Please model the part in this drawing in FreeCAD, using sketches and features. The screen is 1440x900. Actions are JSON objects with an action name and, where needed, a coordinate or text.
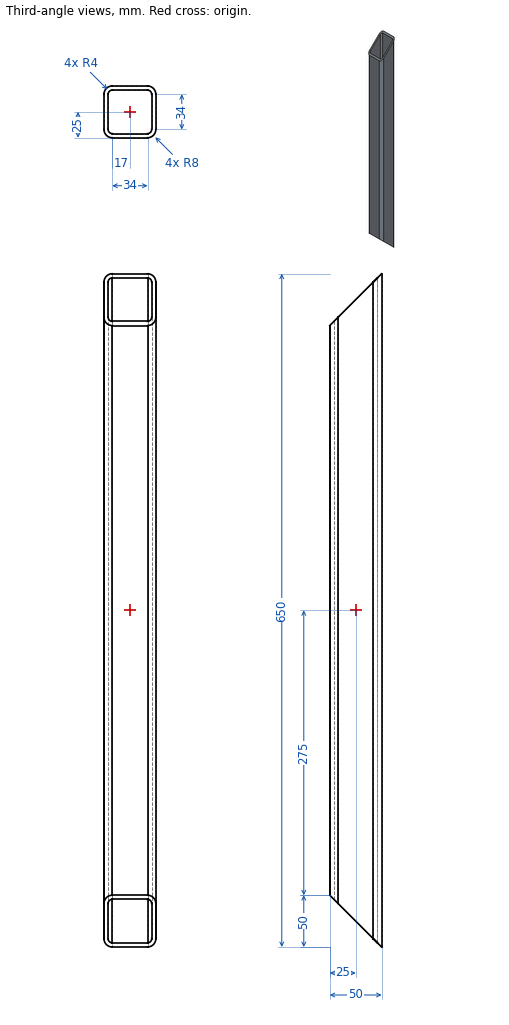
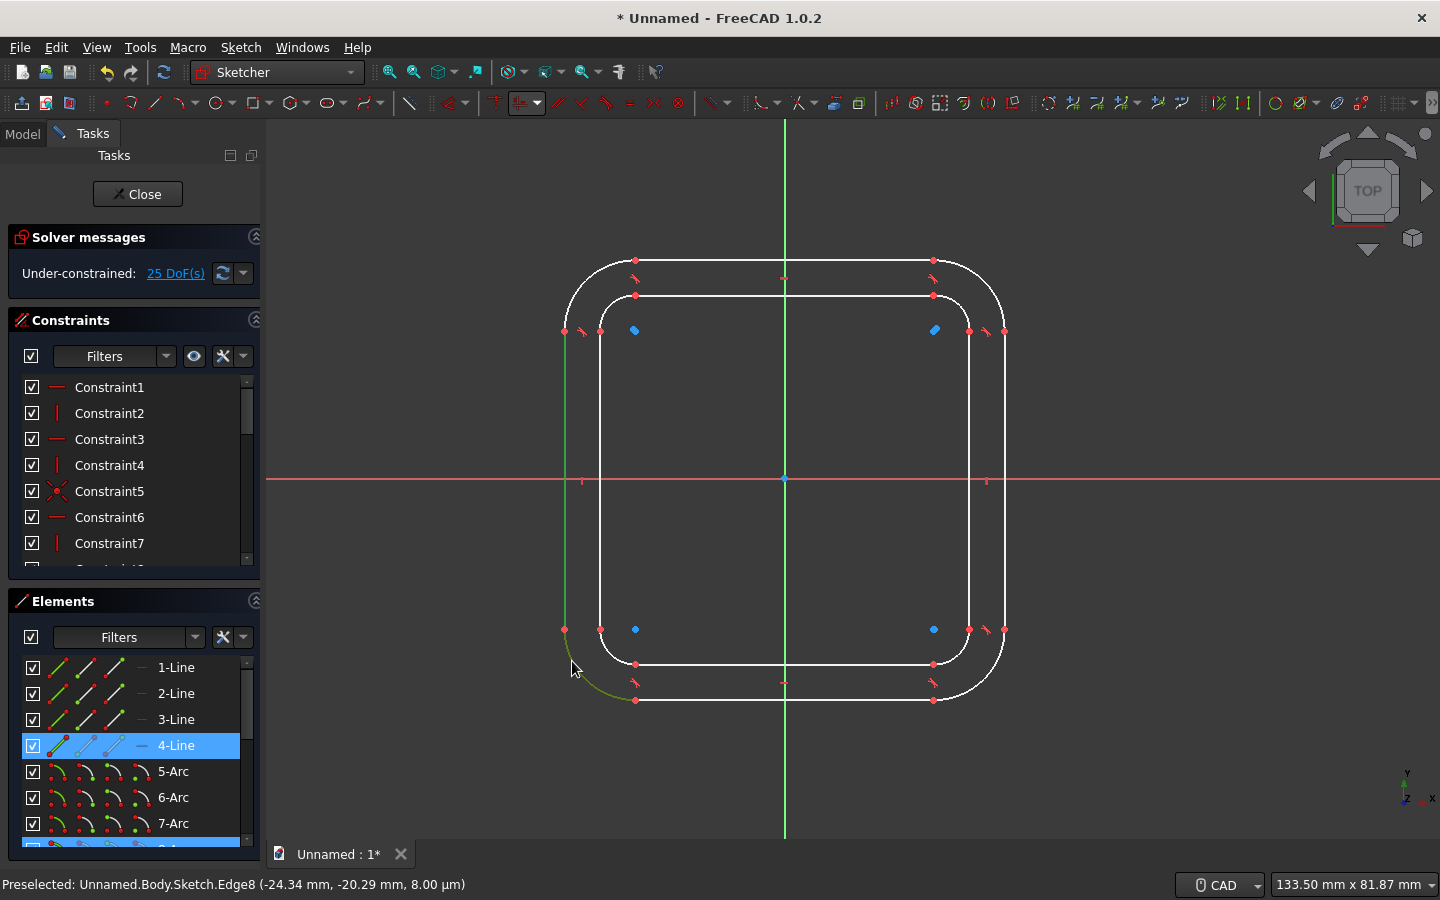
{"action": "left_click", "coordinate": [606, 104]}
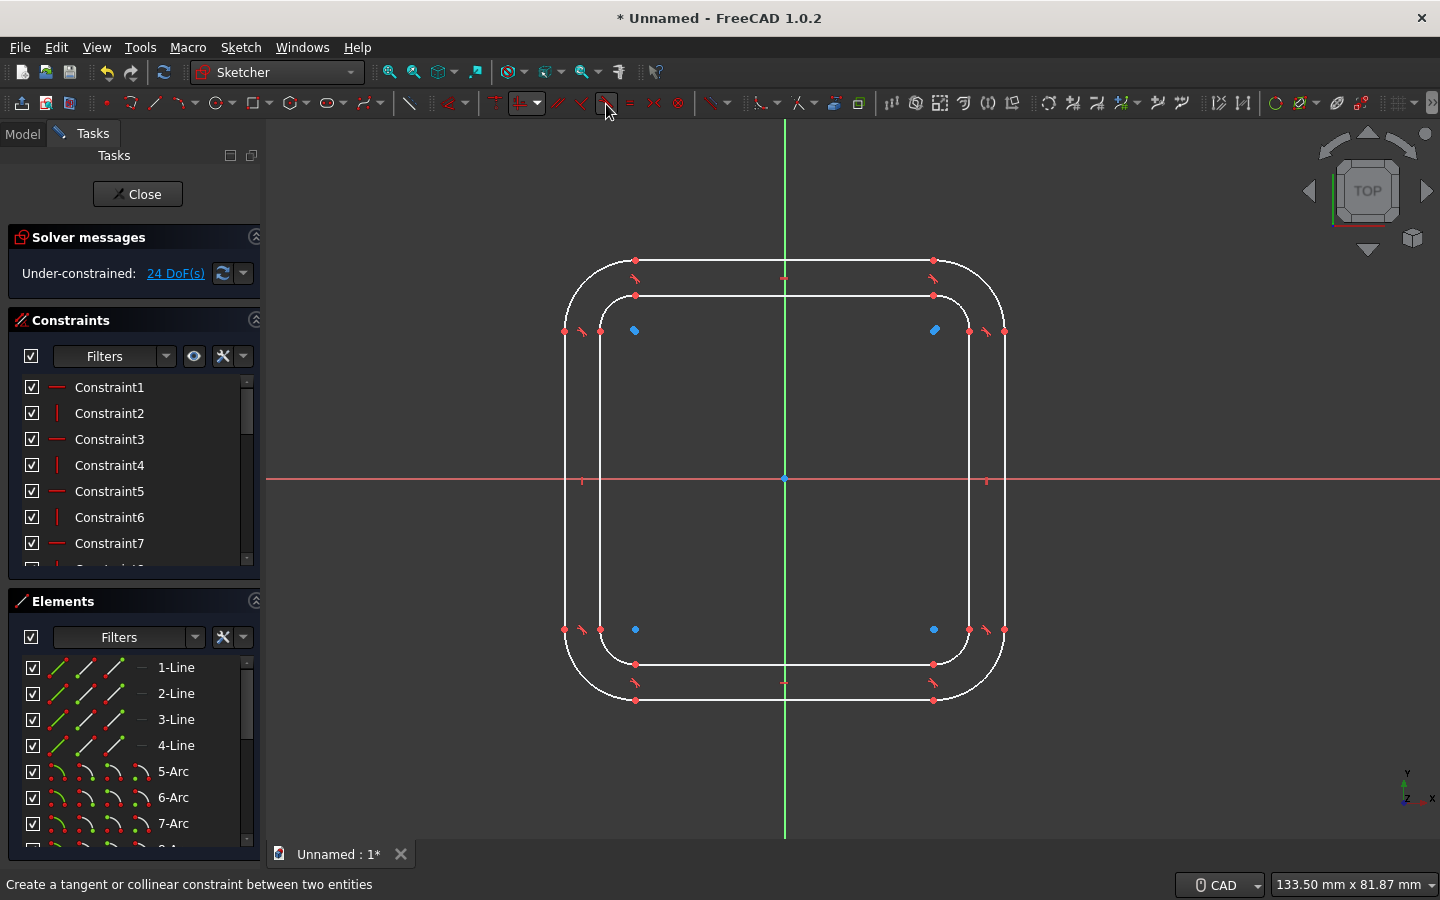
{"action": "left_click", "coordinate": [725, 296]}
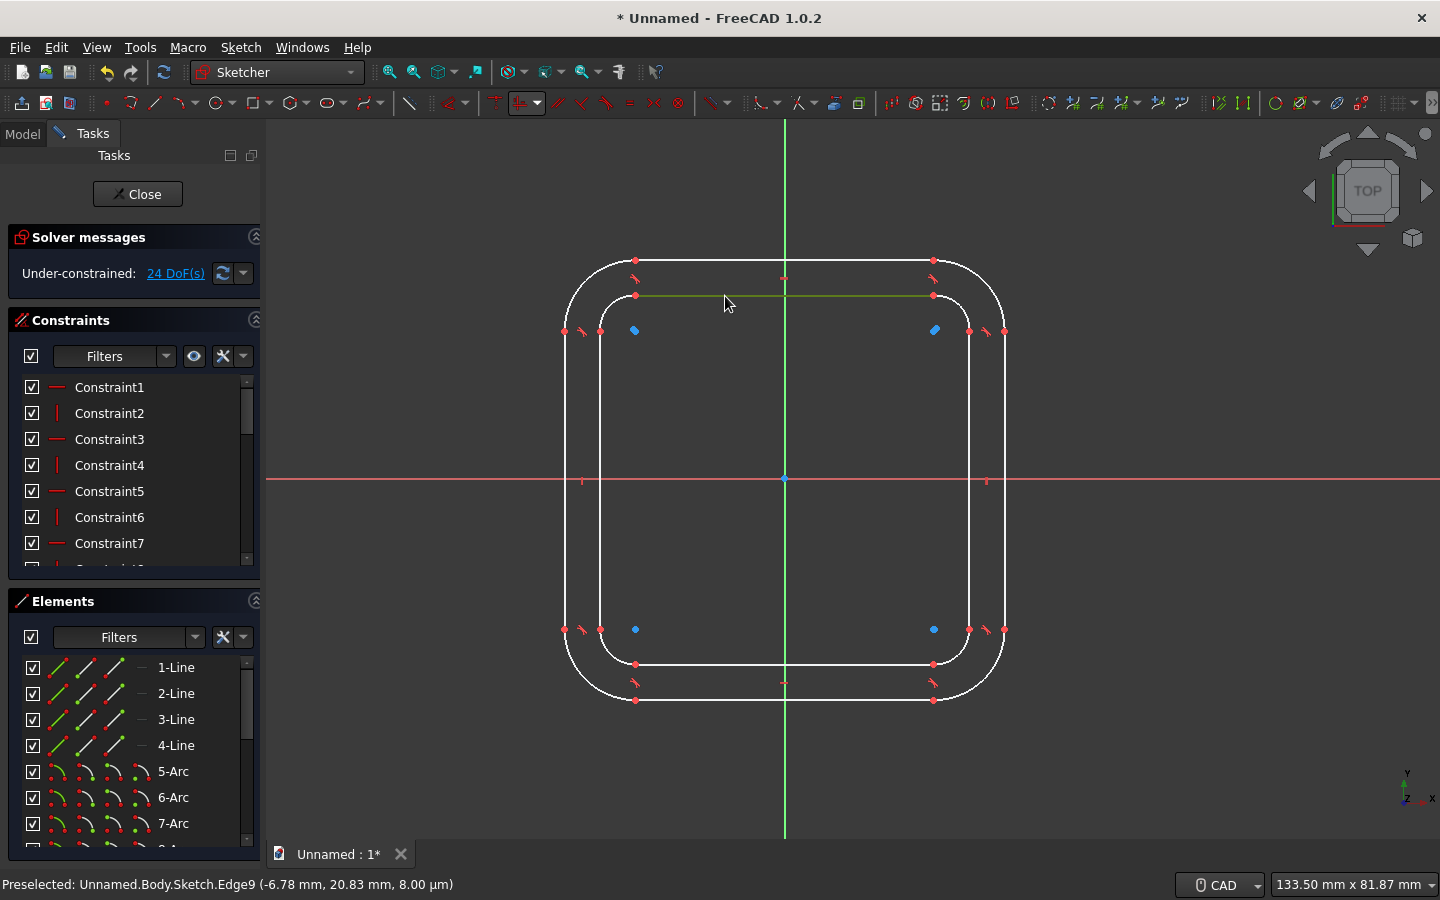
{"action": "left_click", "coordinate": [966, 315]}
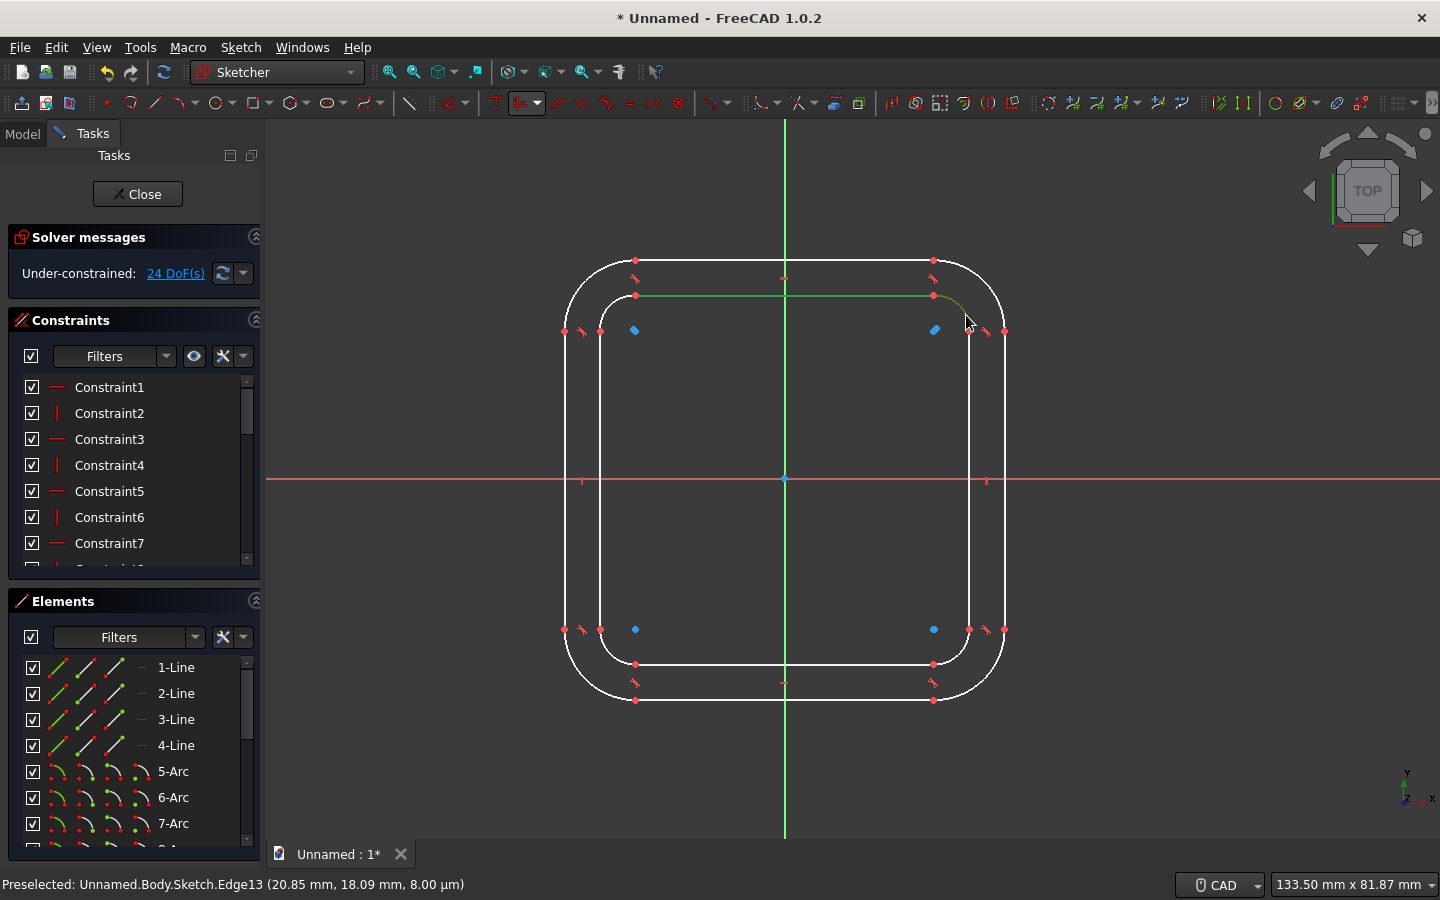
{"action": "left_click", "coordinate": [606, 104]}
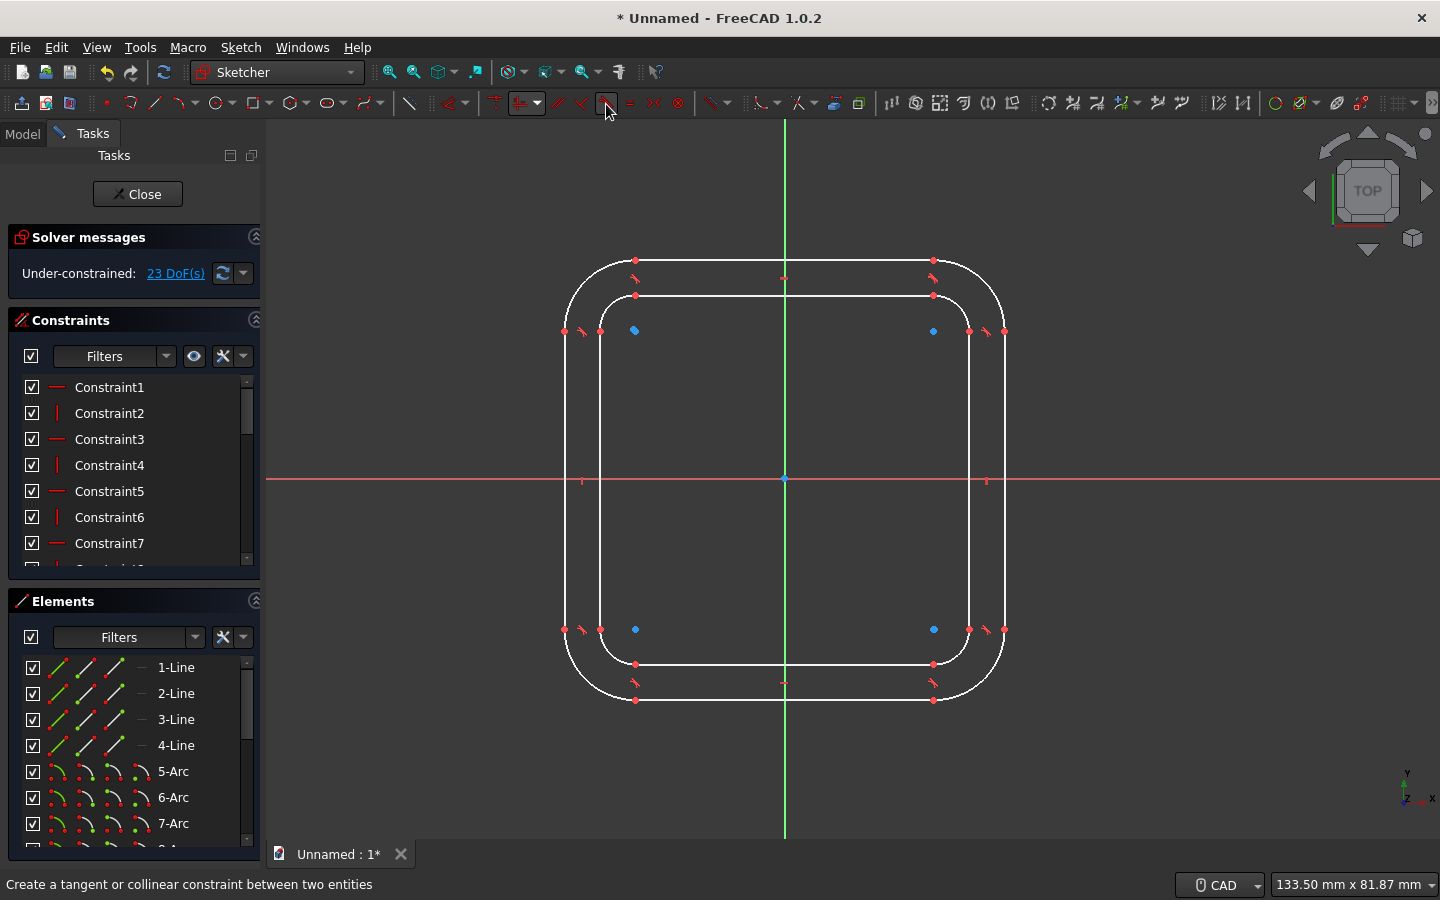
{"action": "left_click", "coordinate": [725, 296]}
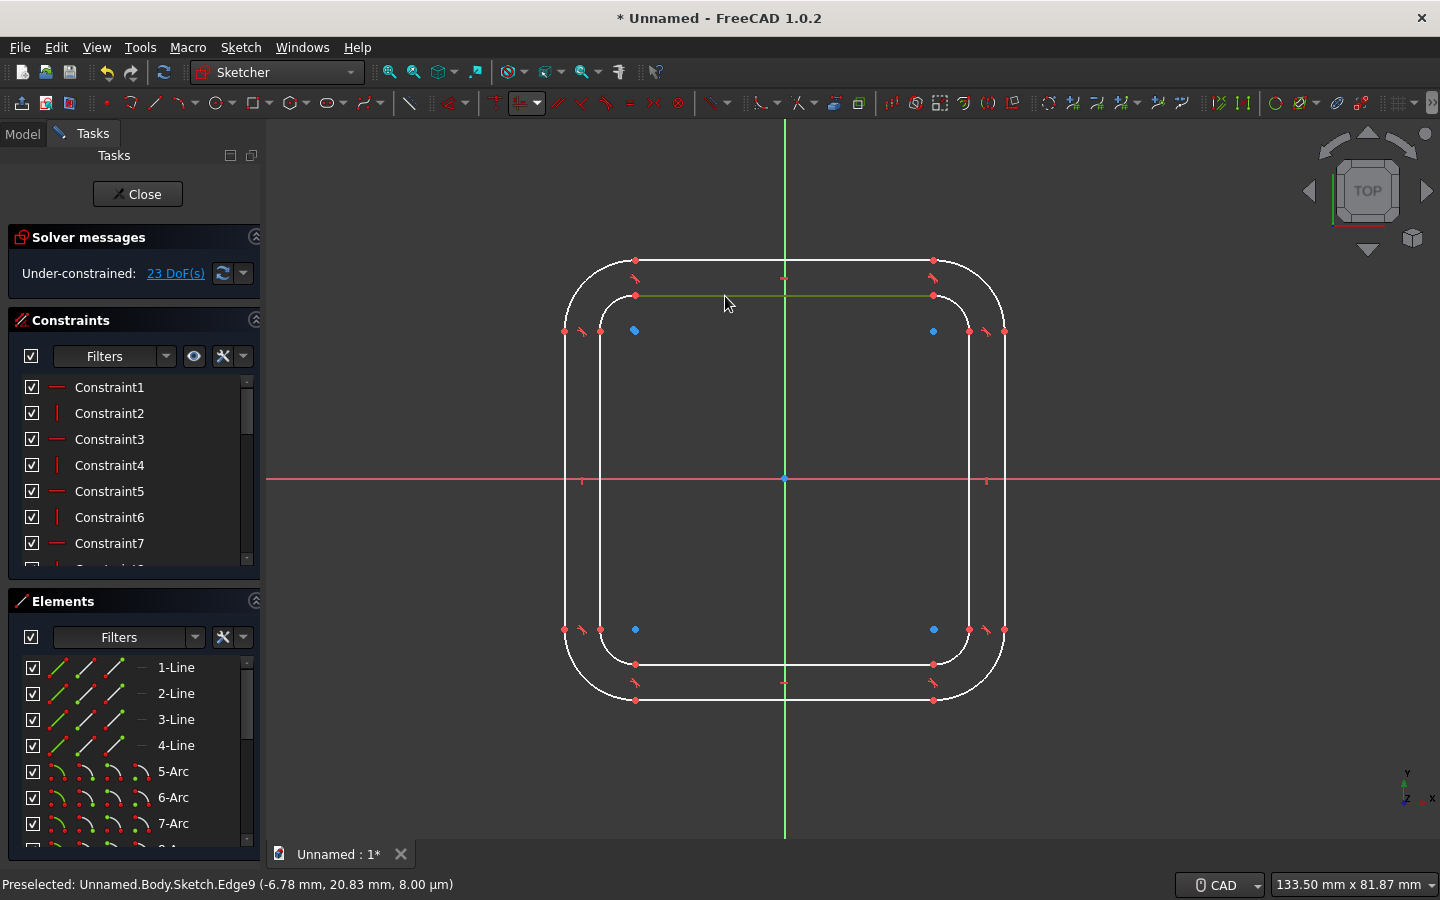
{"action": "left_click", "coordinate": [619, 299]}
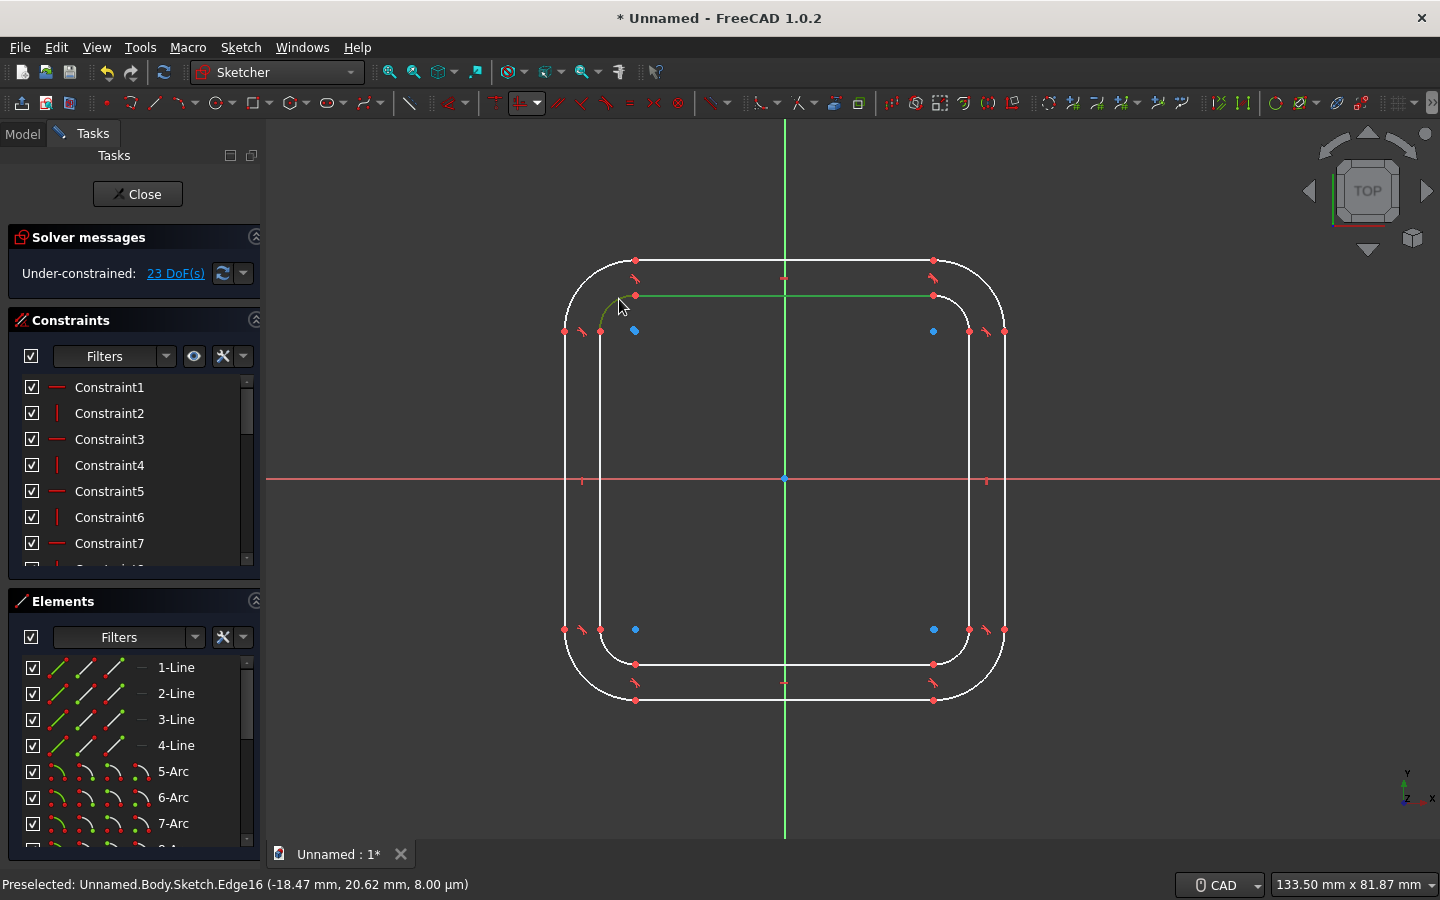
{"action": "left_click", "coordinate": [606, 104]}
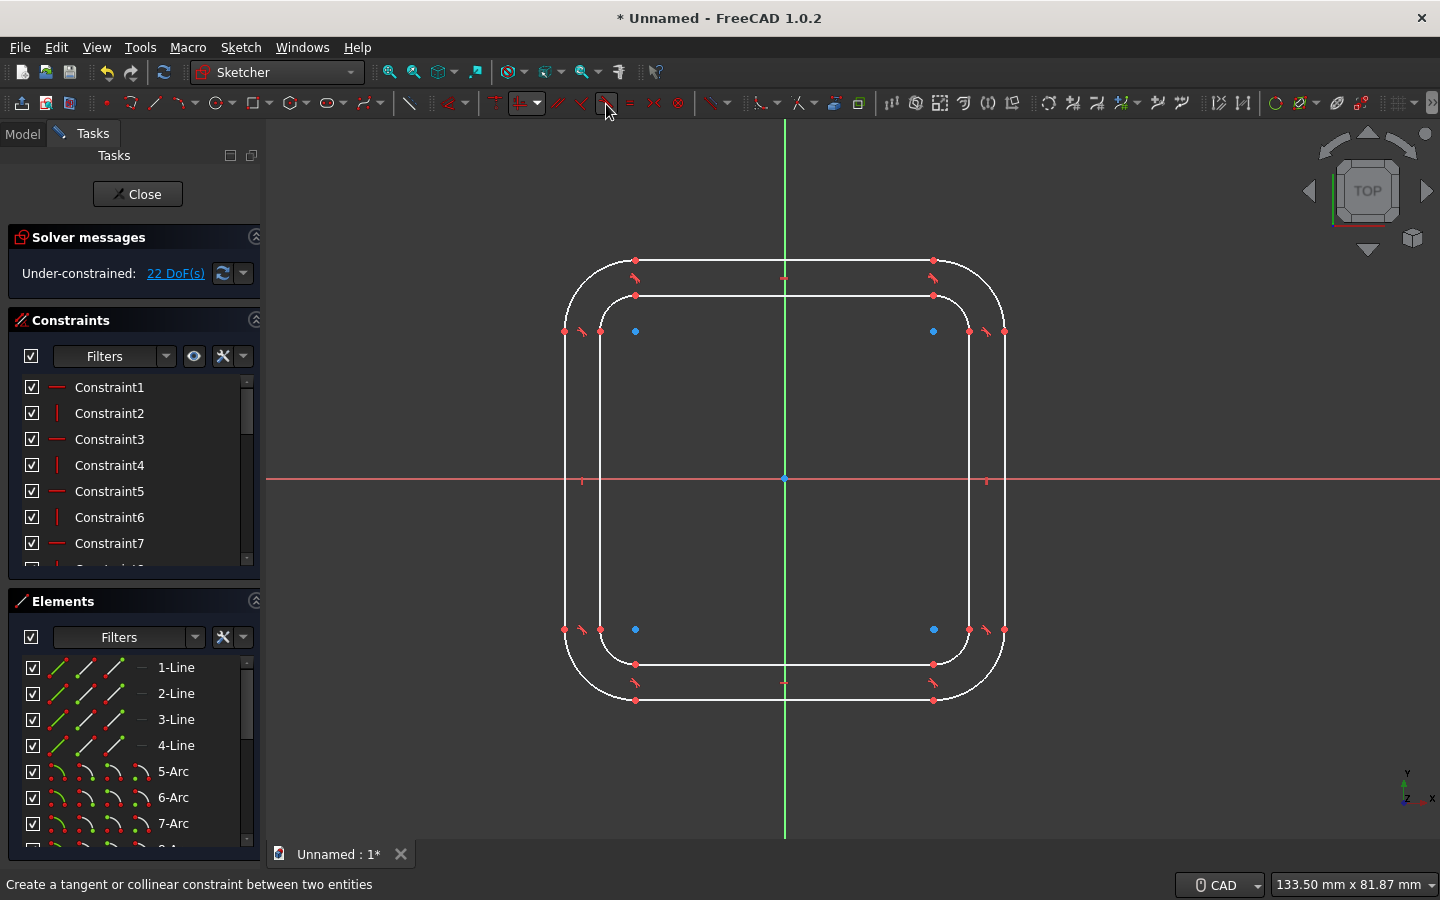
{"action": "left_click", "coordinate": [969, 421]}